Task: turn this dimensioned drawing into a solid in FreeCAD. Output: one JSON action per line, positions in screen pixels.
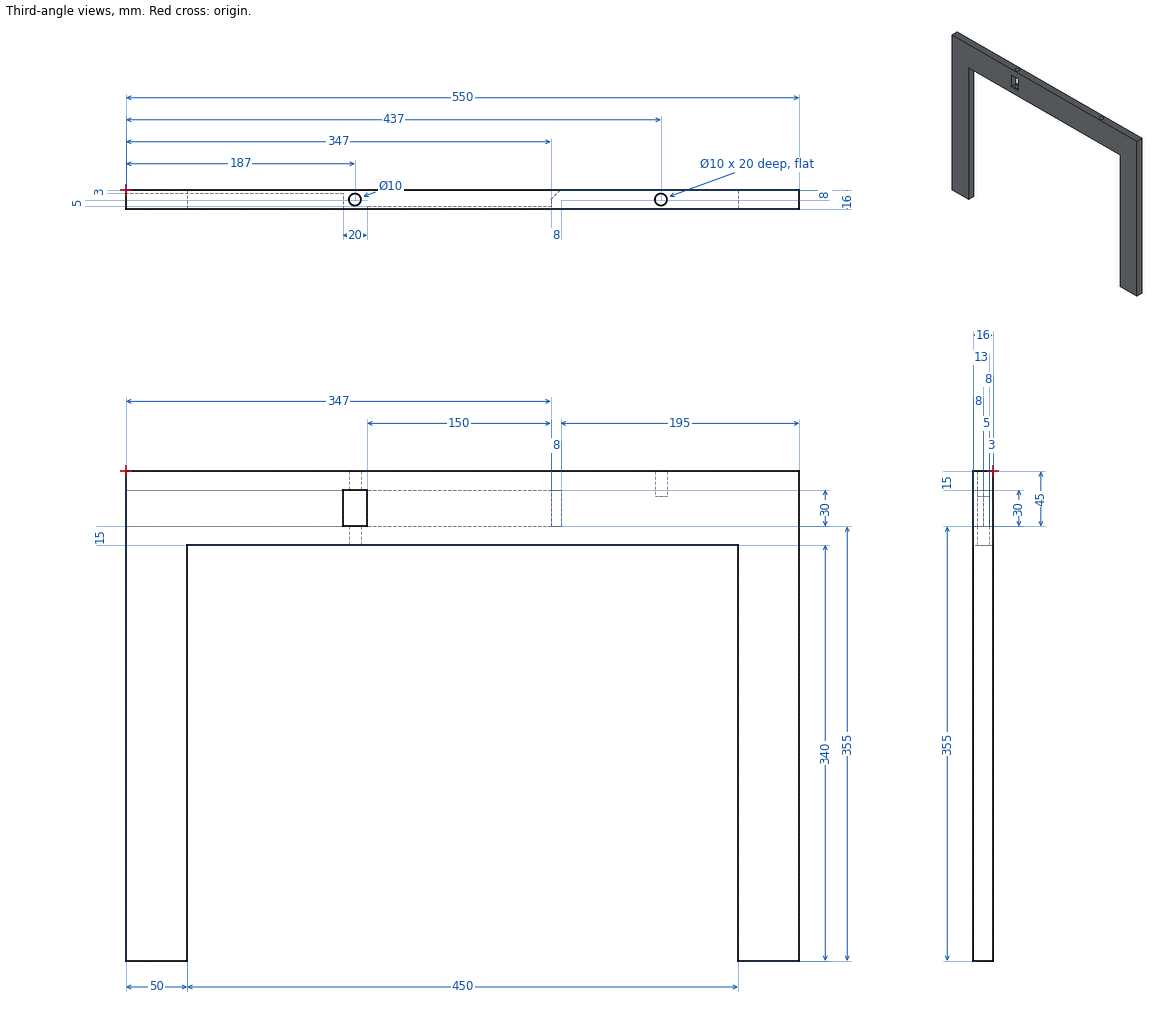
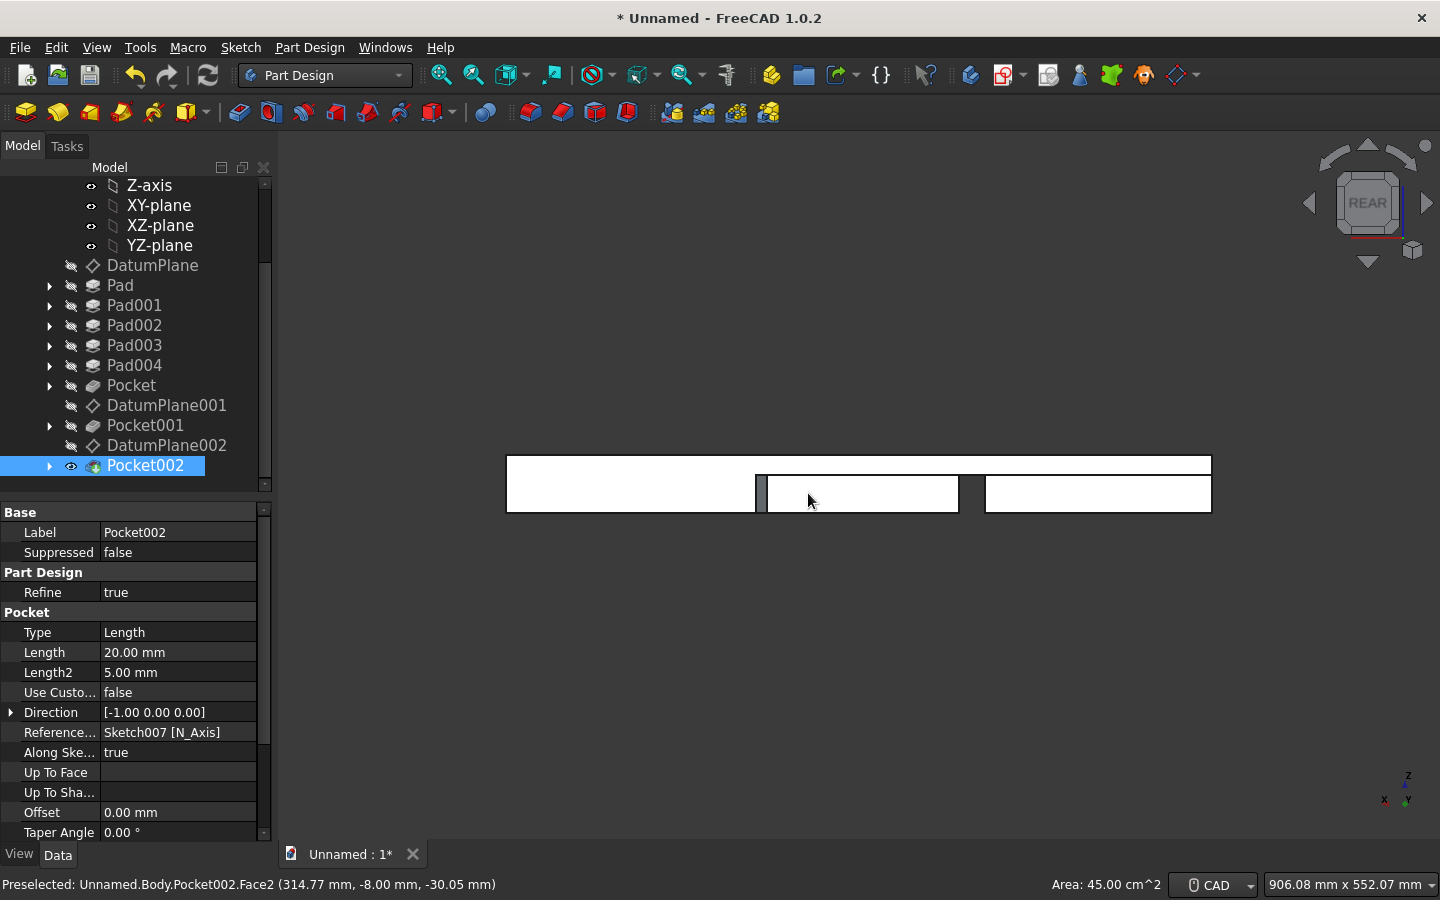
{"action": "left_click", "coordinate": [1004, 76]}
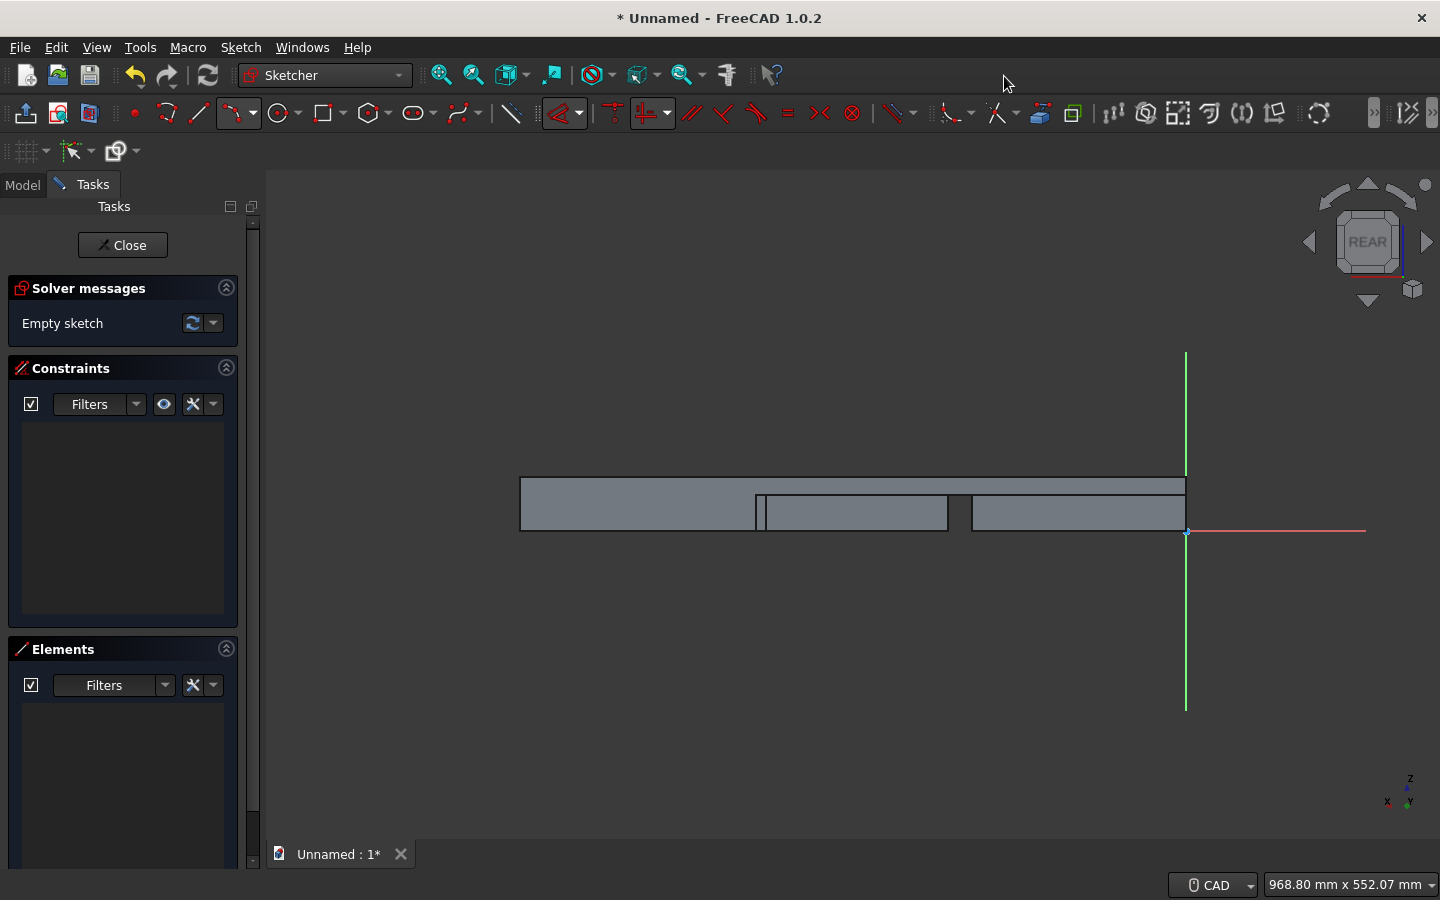
{"action": "scroll", "coordinate": [1275, 530], "scroll_direction": "up", "scroll_amount": 2}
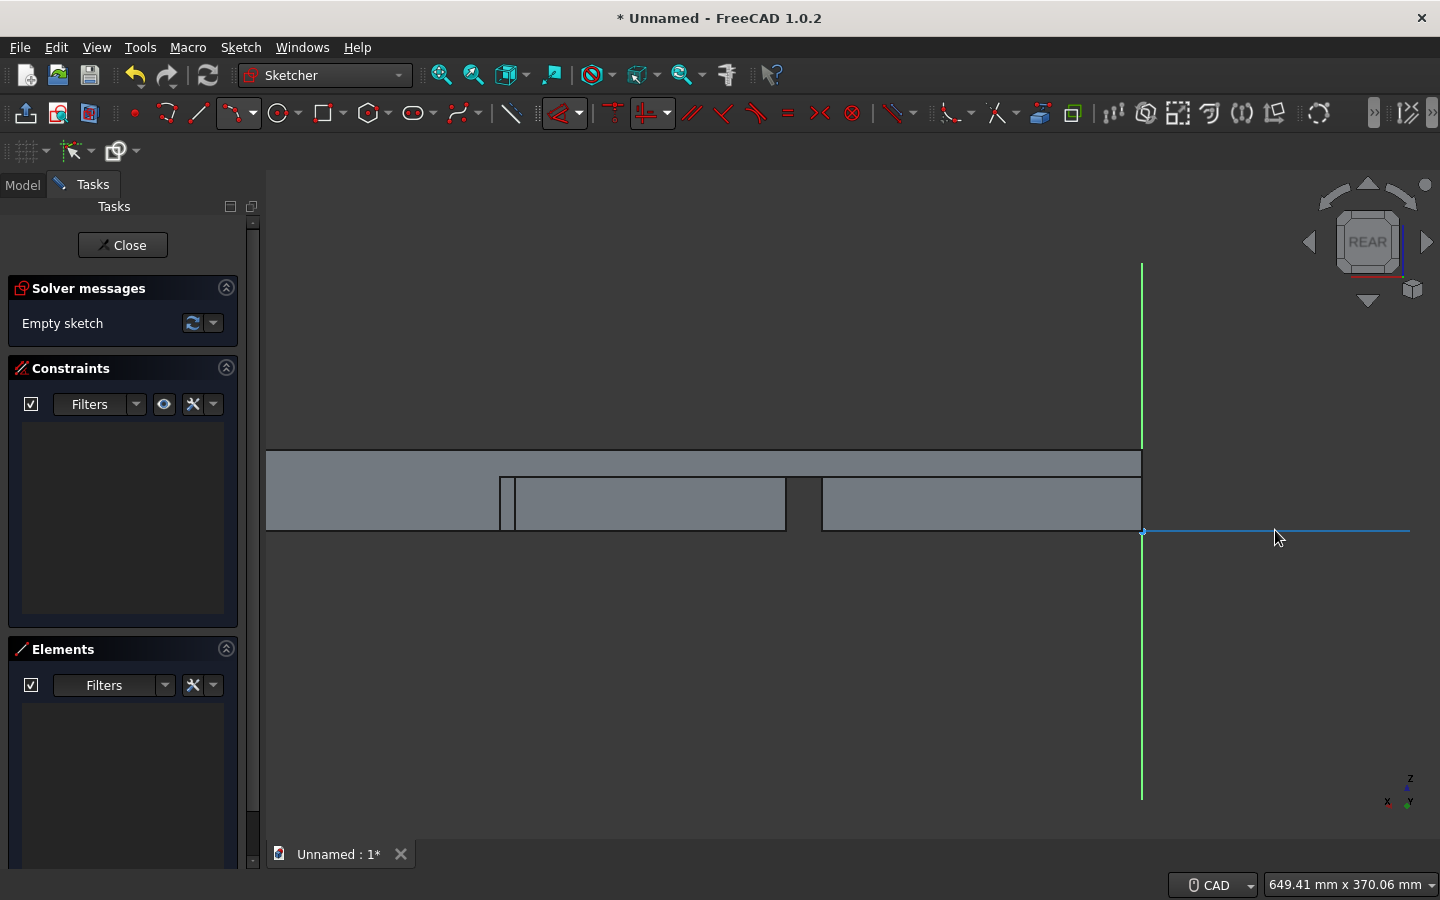
{"action": "left_click", "coordinate": [324, 114]}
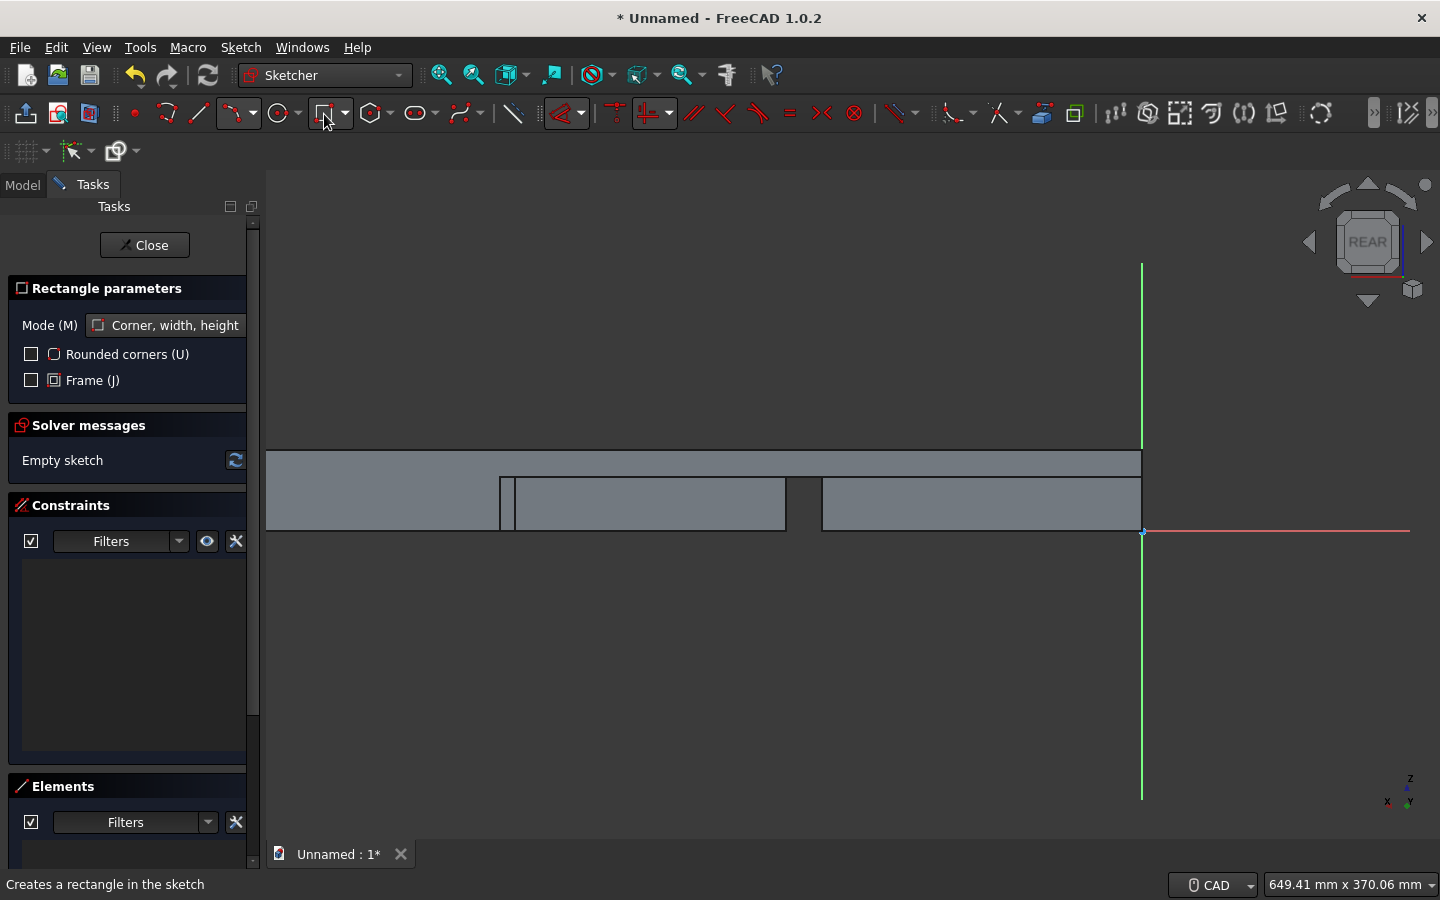
{"action": "left_click", "coordinate": [515, 477]}
{"action": "left_click", "coordinate": [786, 531]}
{"action": "key", "text": "Escape"}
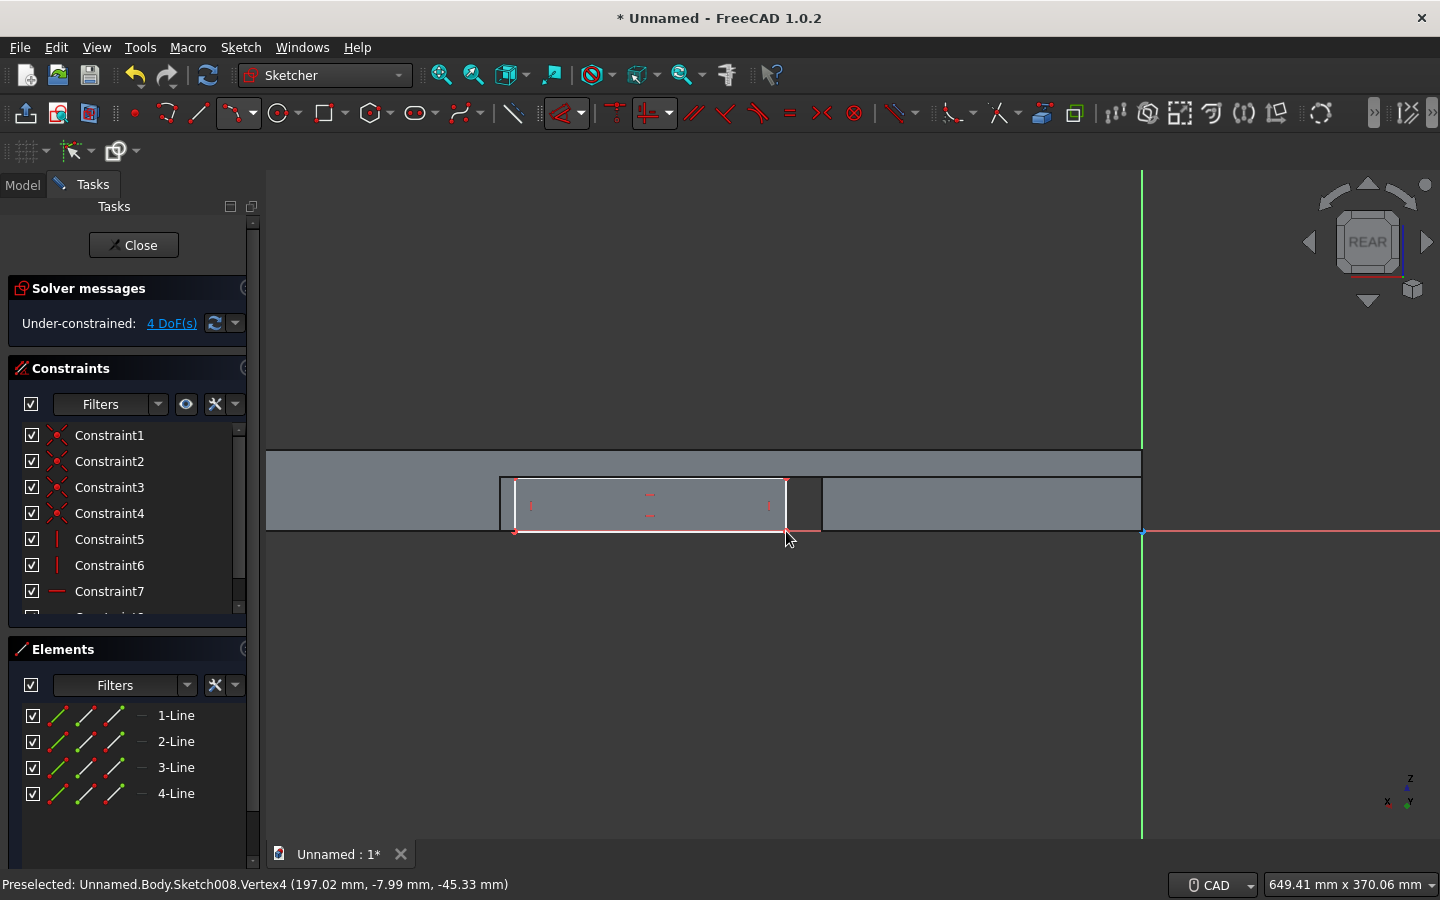
{"action": "left_click", "coordinate": [515, 532]}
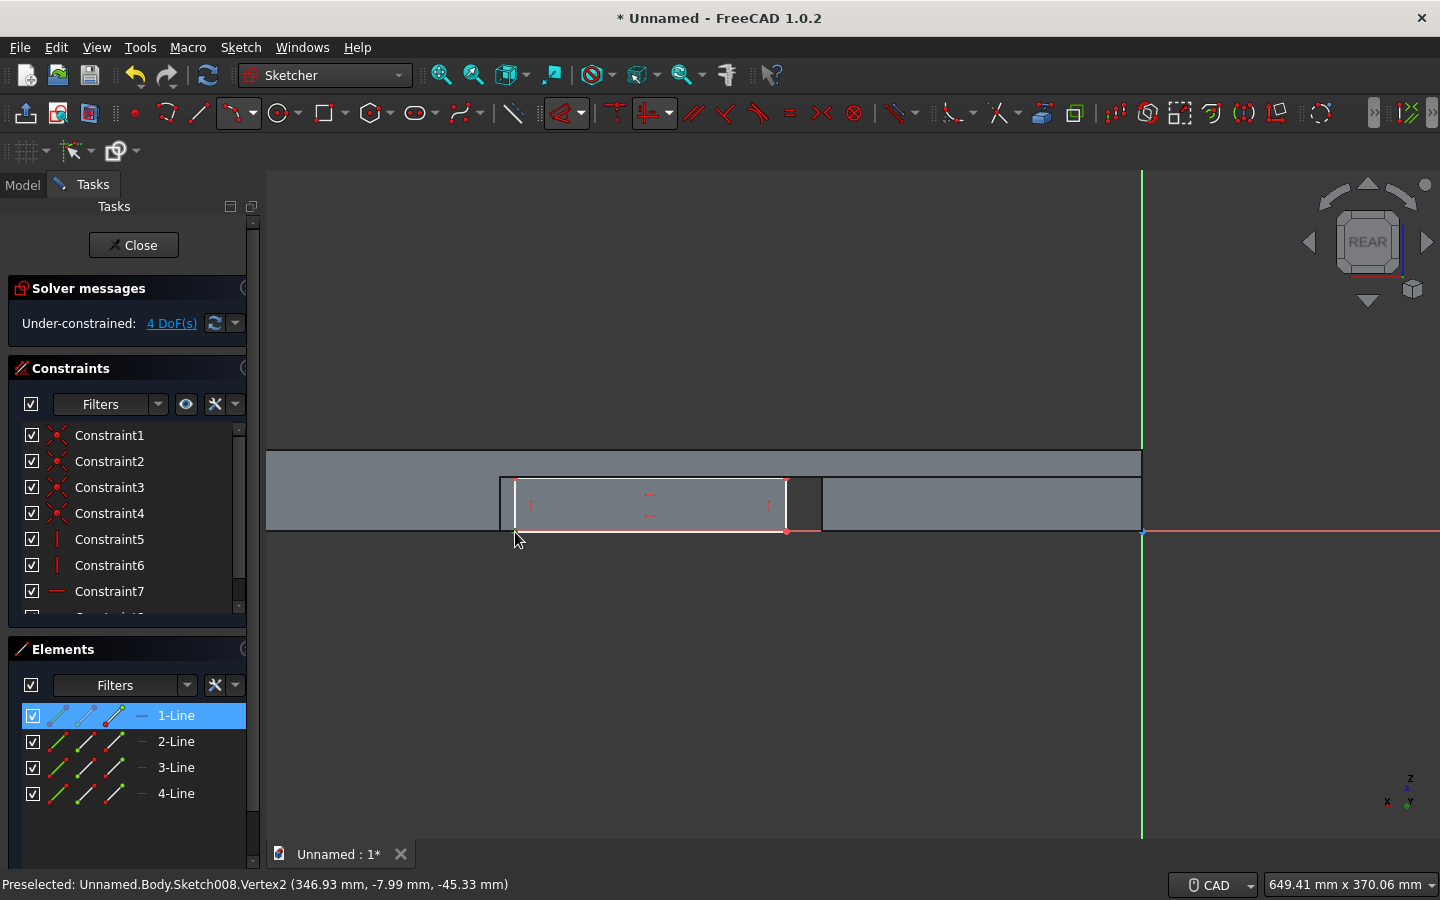
{"action": "left_click", "coordinate": [434, 531]}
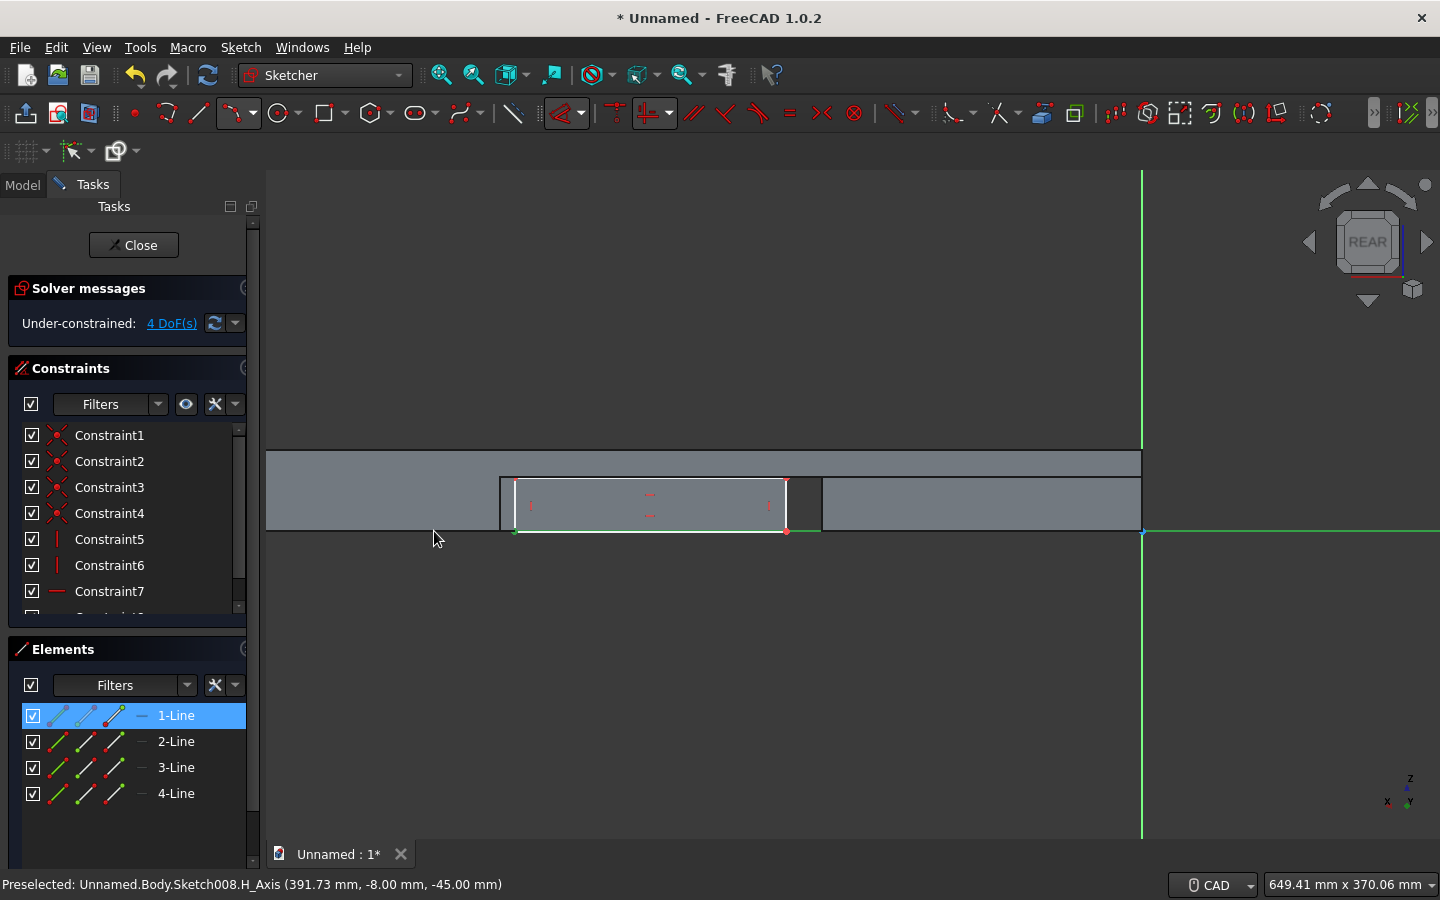
{"action": "left_click", "coordinate": [616, 114]}